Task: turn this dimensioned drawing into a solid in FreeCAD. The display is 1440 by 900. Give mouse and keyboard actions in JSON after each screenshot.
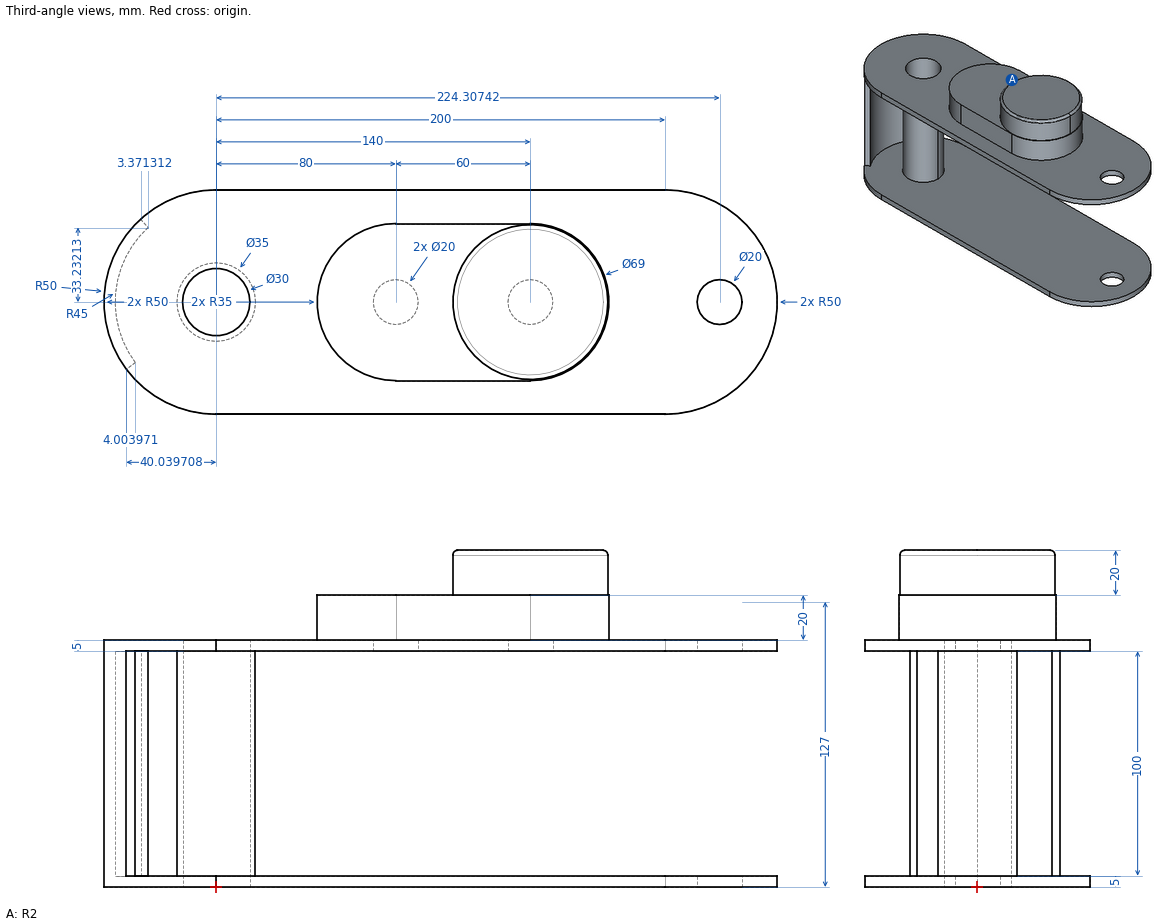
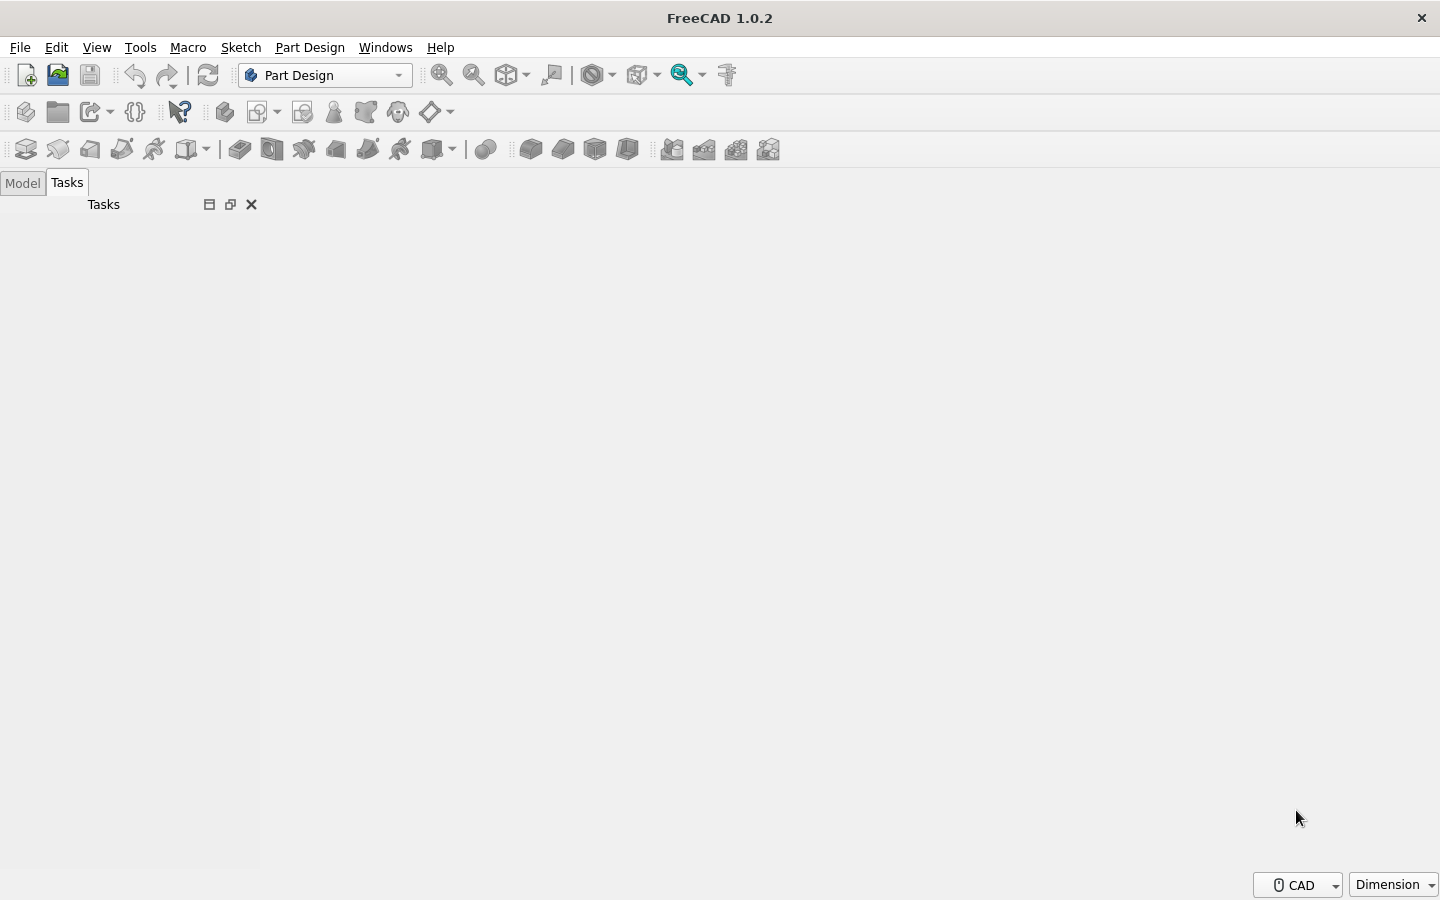
{"action": "left_click", "coordinate": [26, 76]}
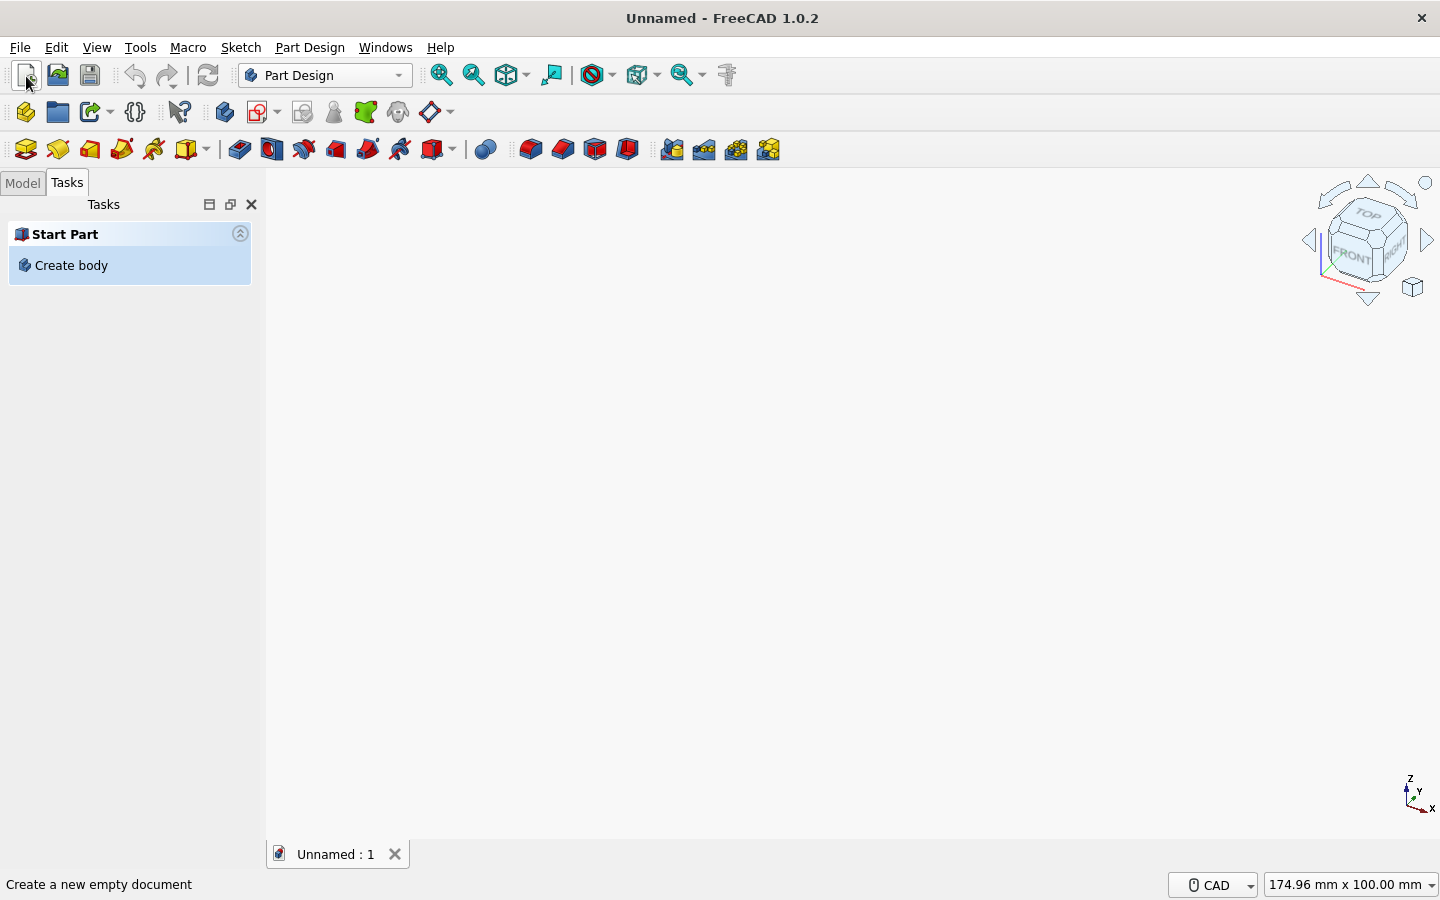
{"action": "left_click", "coordinate": [258, 112]}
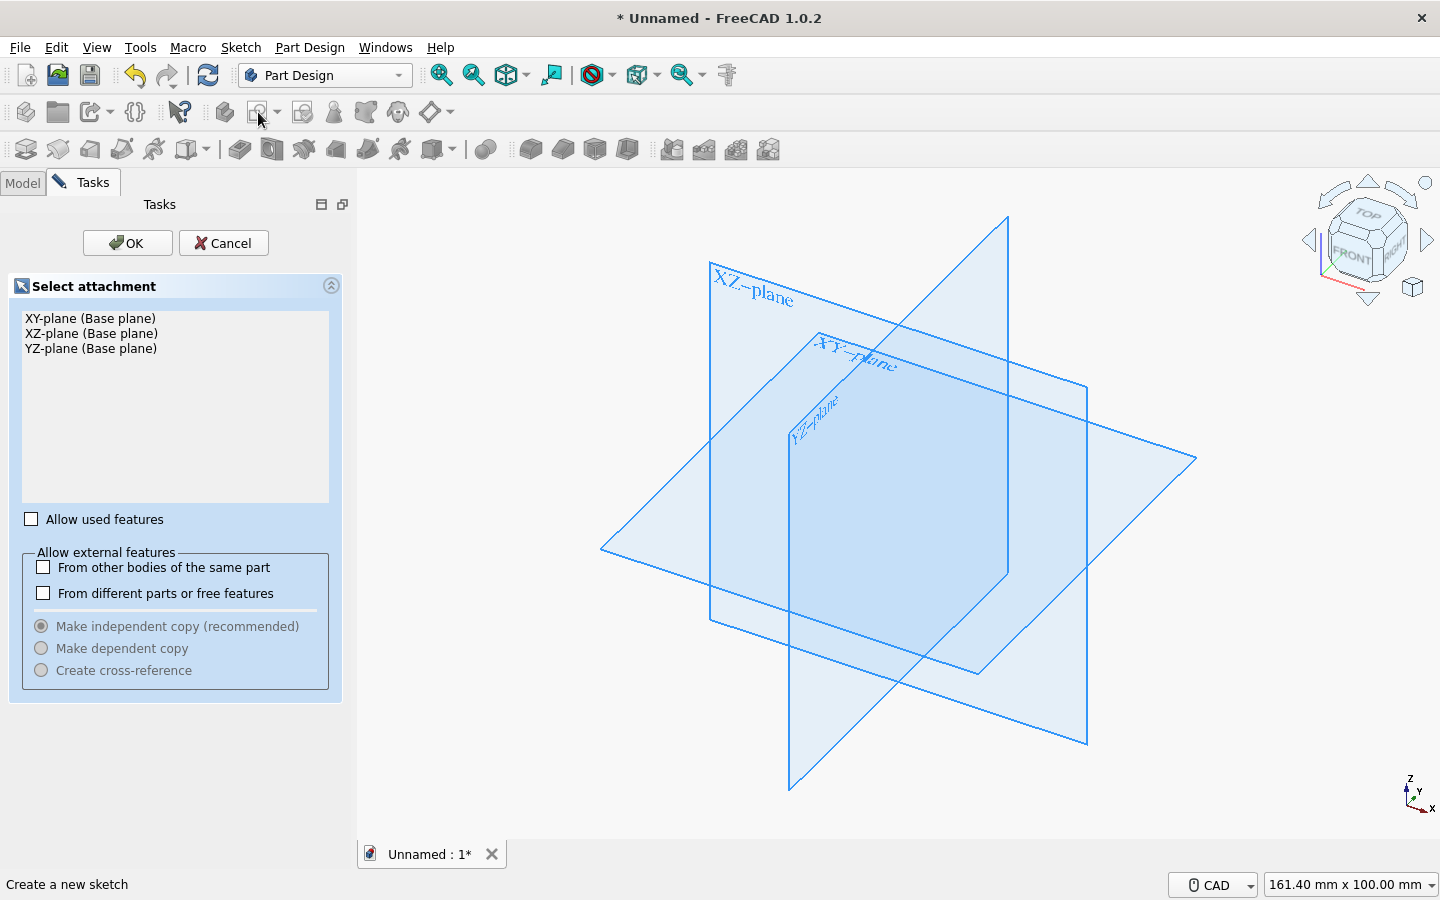
{"action": "left_click", "coordinate": [82, 318]}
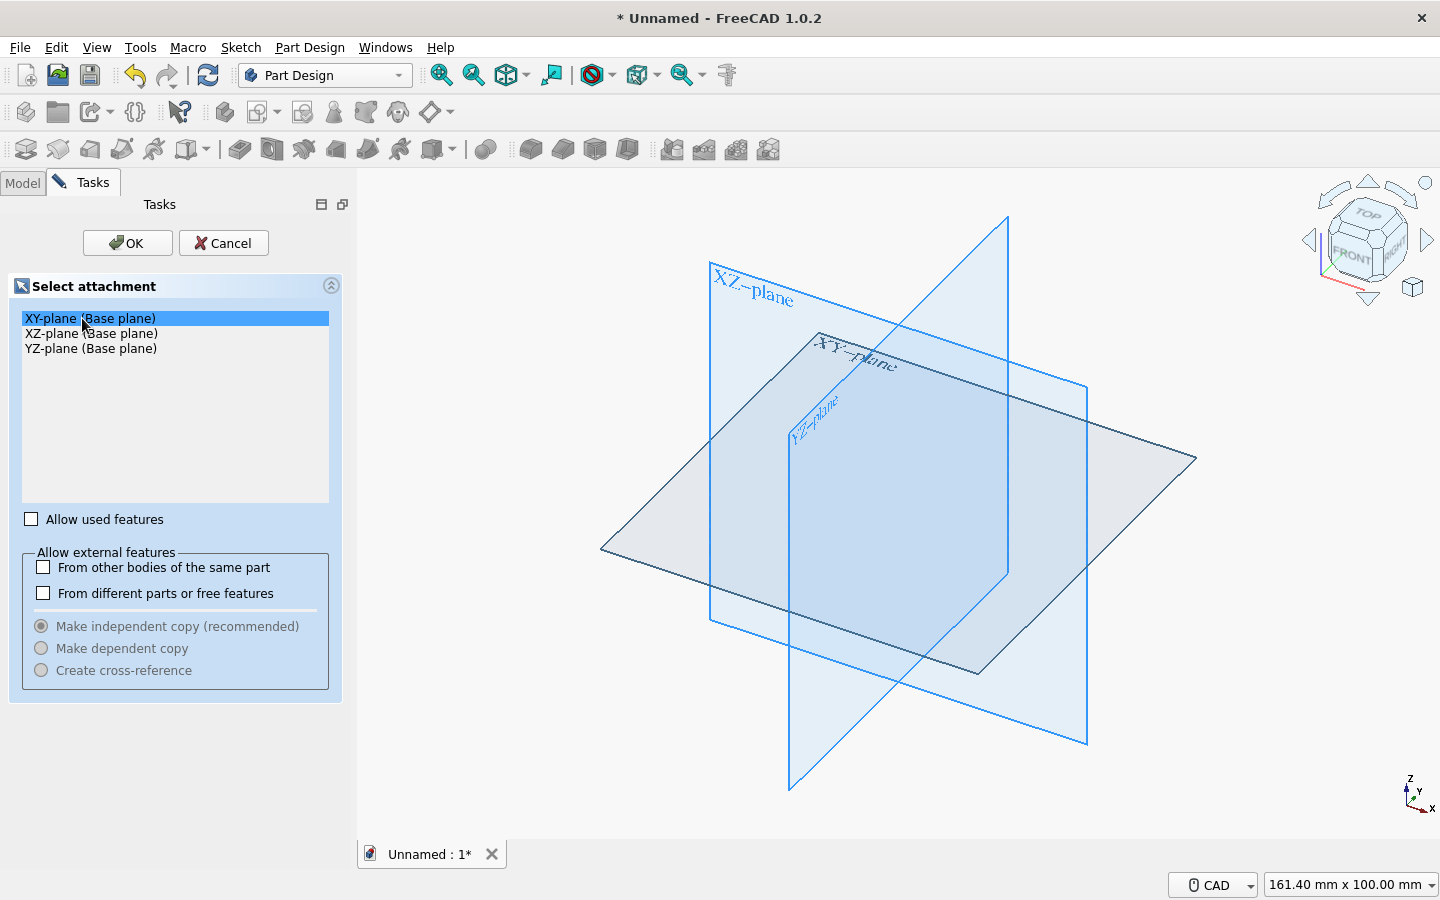
{"action": "left_click", "coordinate": [128, 243]}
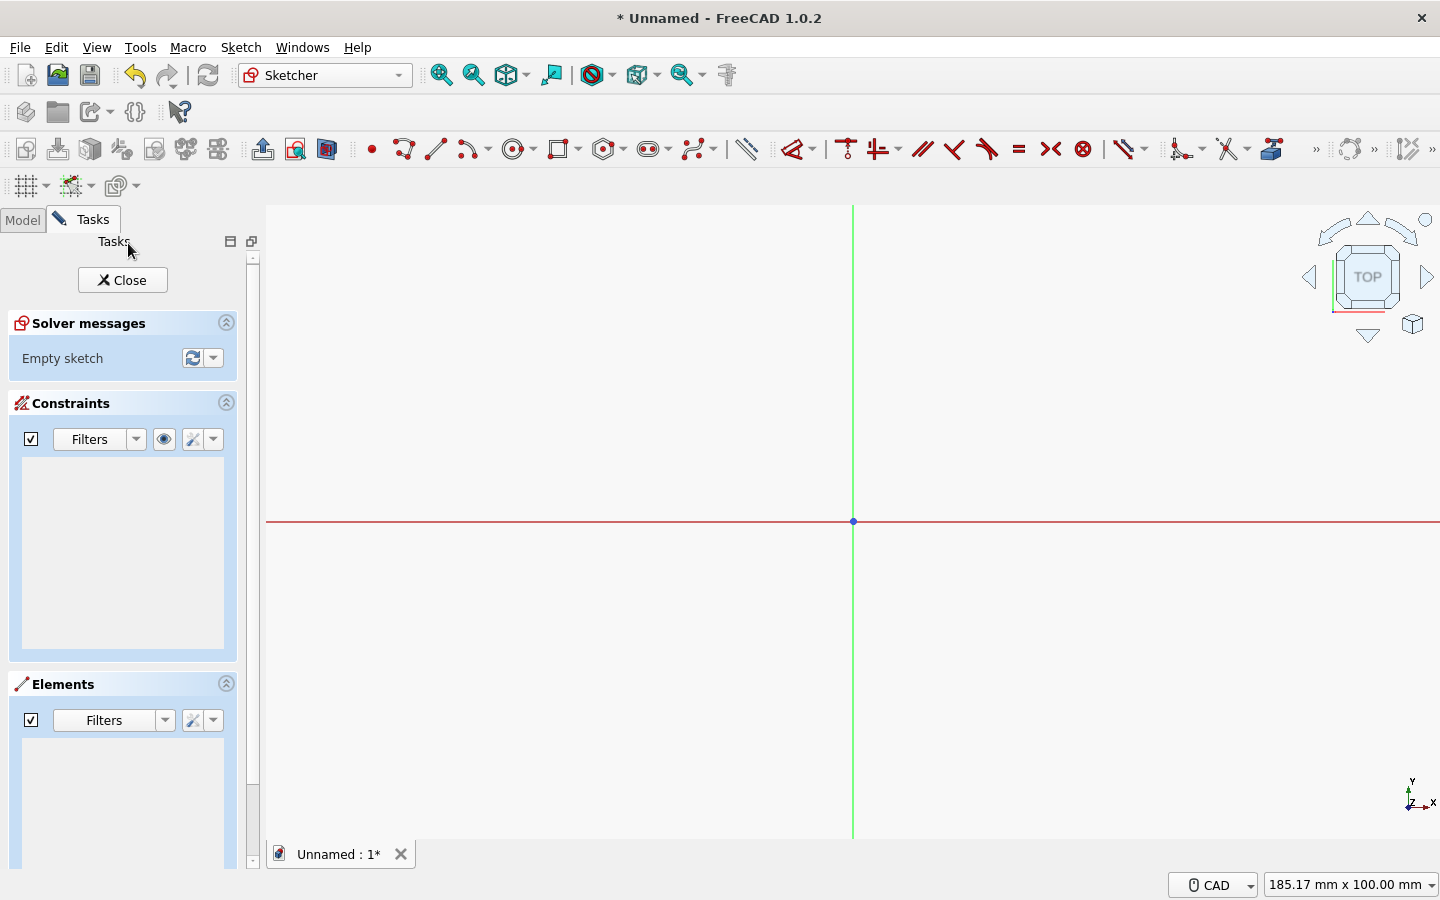
{"action": "scroll", "coordinate": [376, 522], "scroll_direction": "down", "scroll_amount": 5}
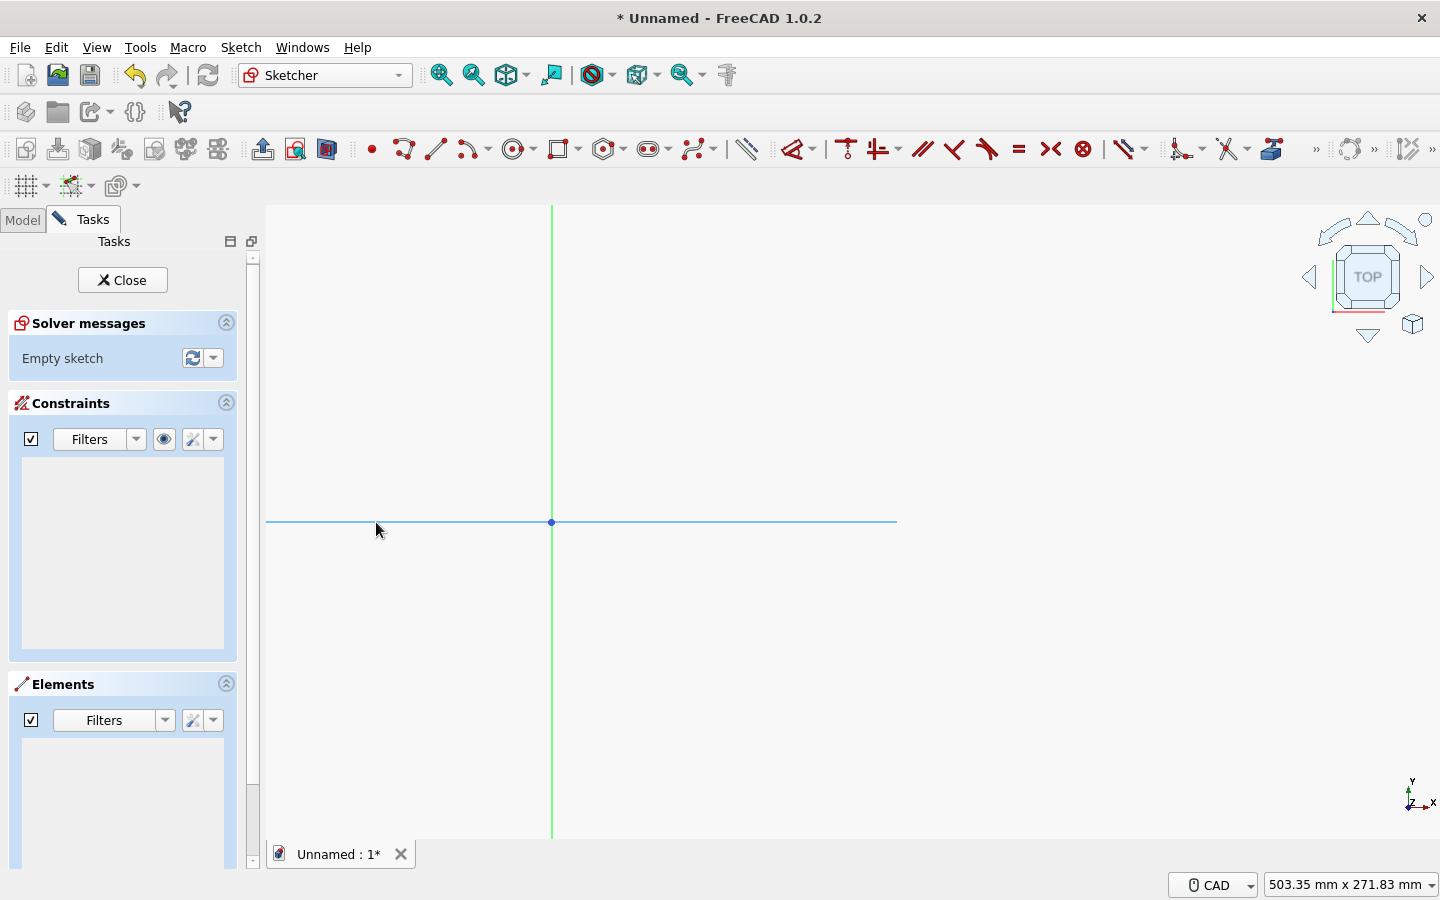
{"action": "left_click", "coordinate": [648, 150]}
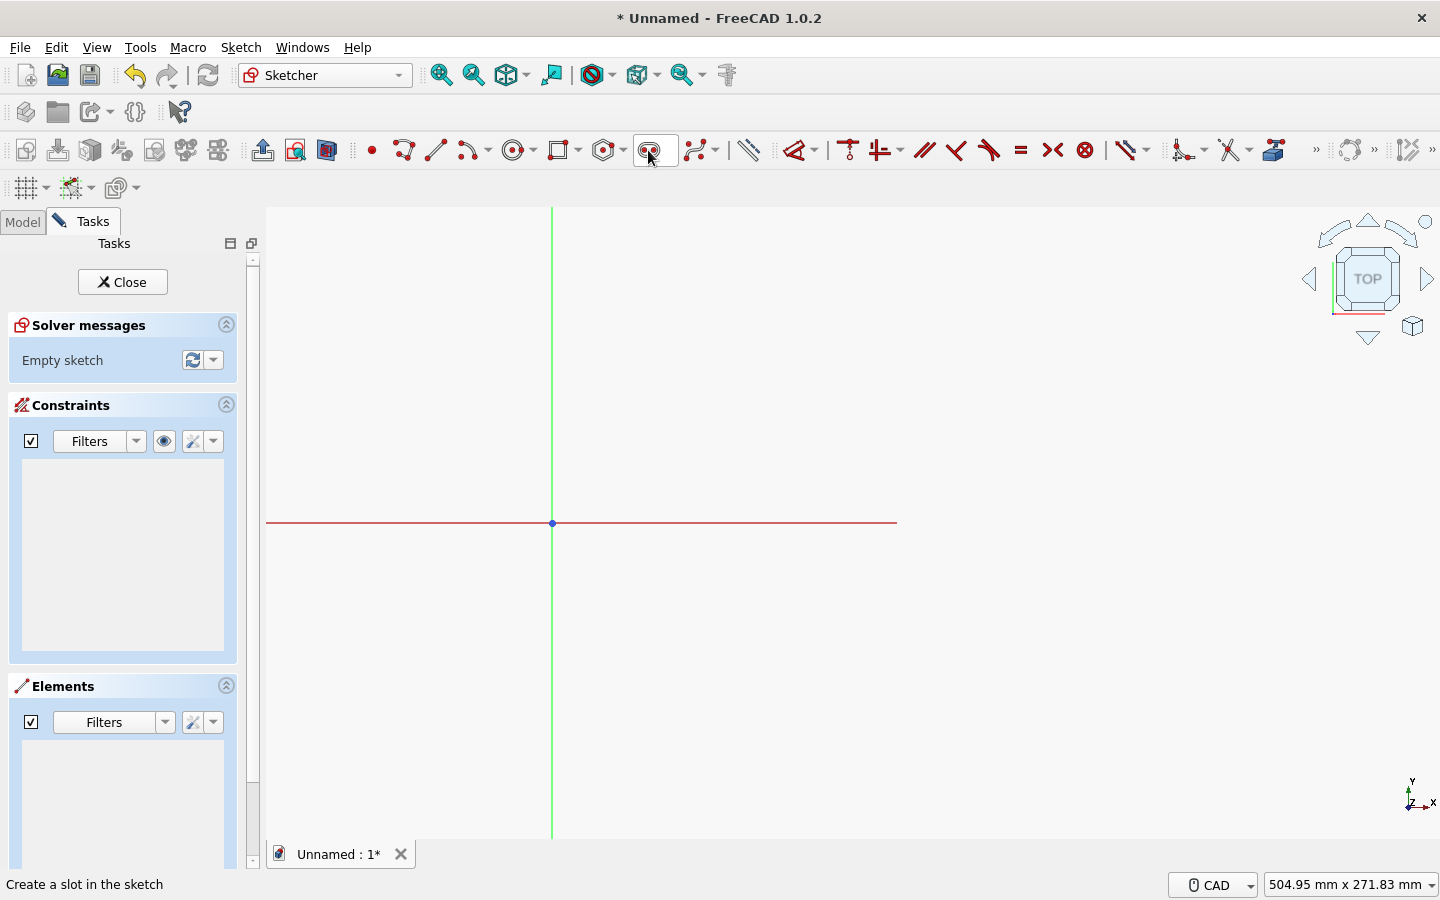
{"action": "left_click", "coordinate": [552, 523]}